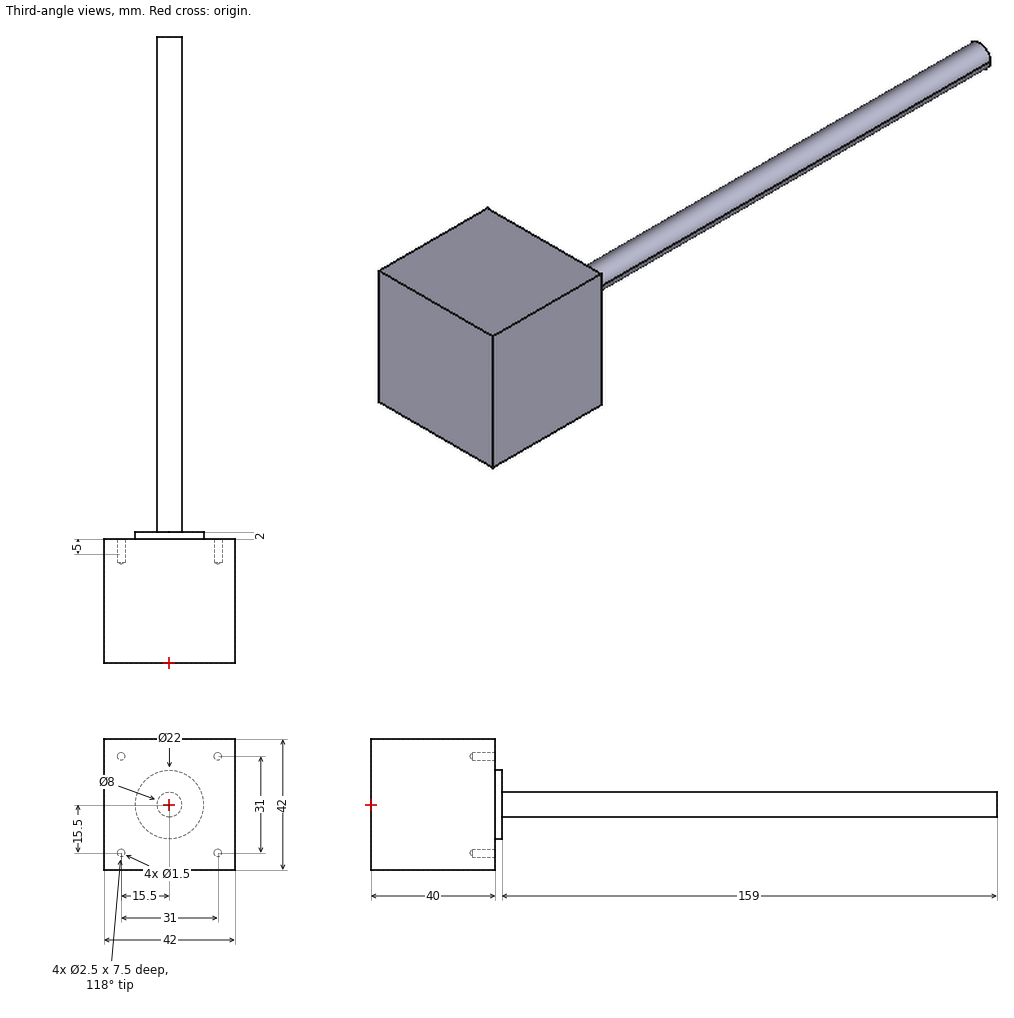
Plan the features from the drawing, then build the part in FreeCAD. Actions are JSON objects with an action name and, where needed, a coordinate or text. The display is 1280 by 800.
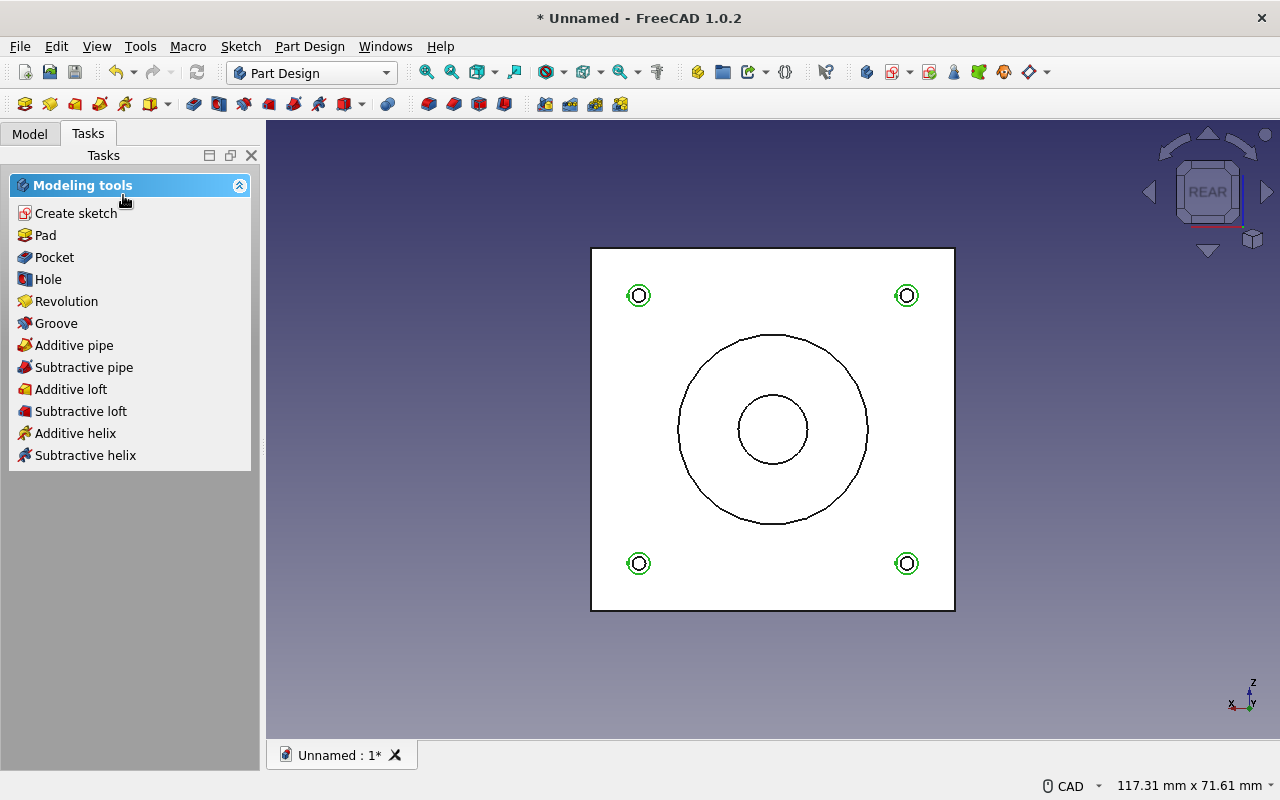
{"action": "left_click", "coordinate": [219, 104]}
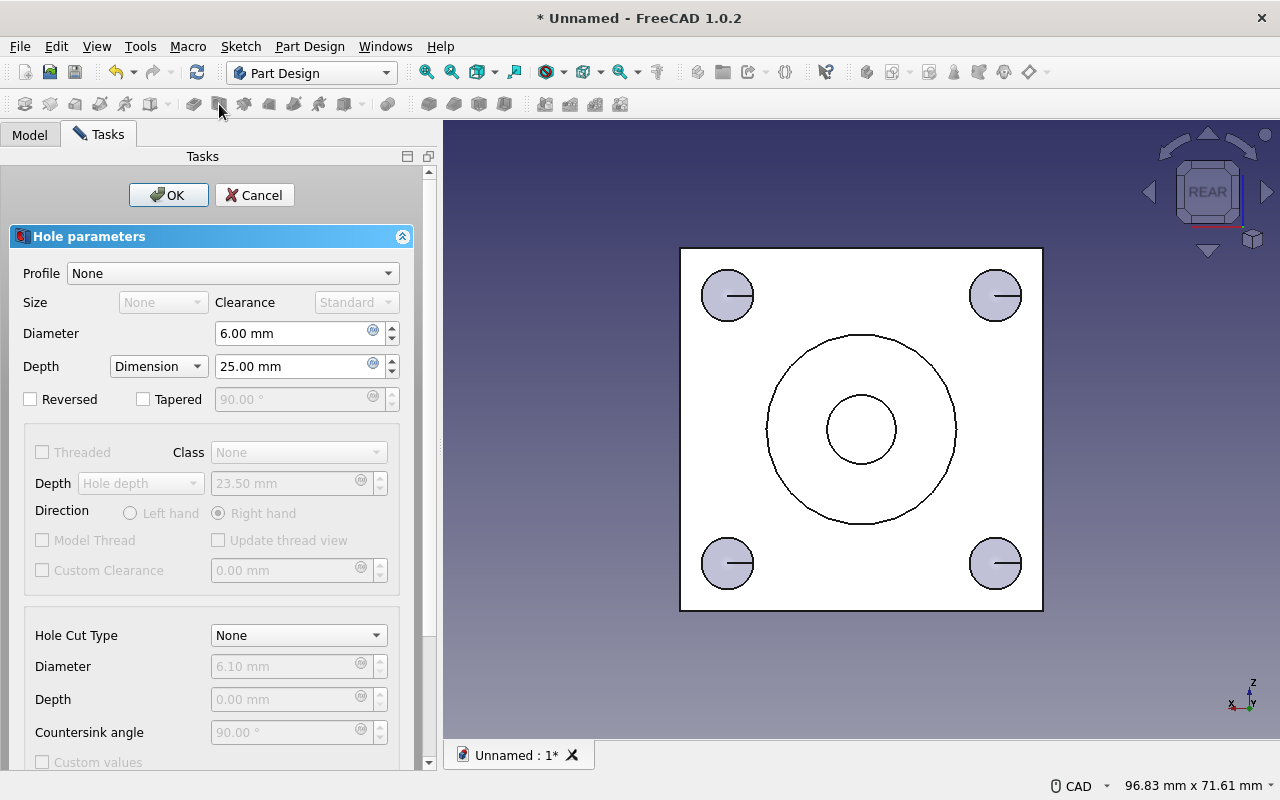
{"action": "triple_click", "coordinate": [300, 334]}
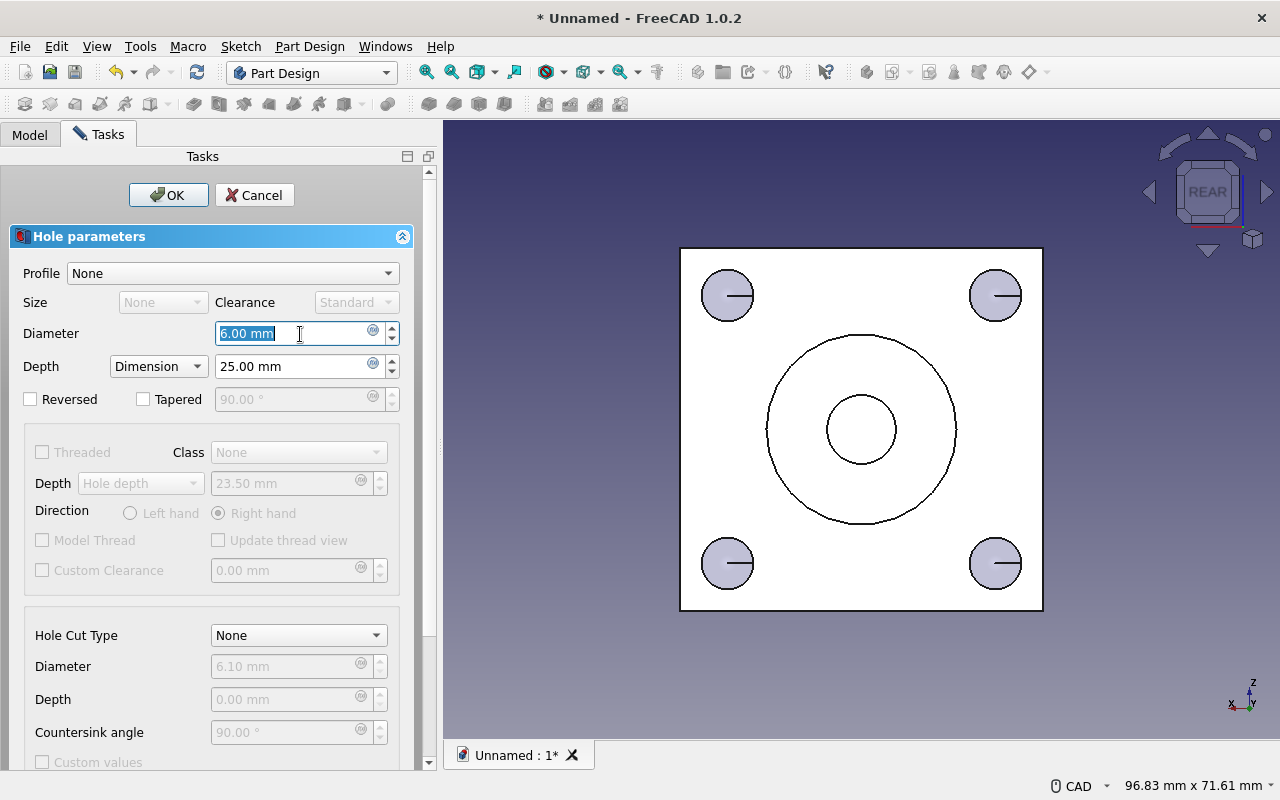
{"action": "type", "text": "2.5"}
{"action": "key", "text": "Tab"}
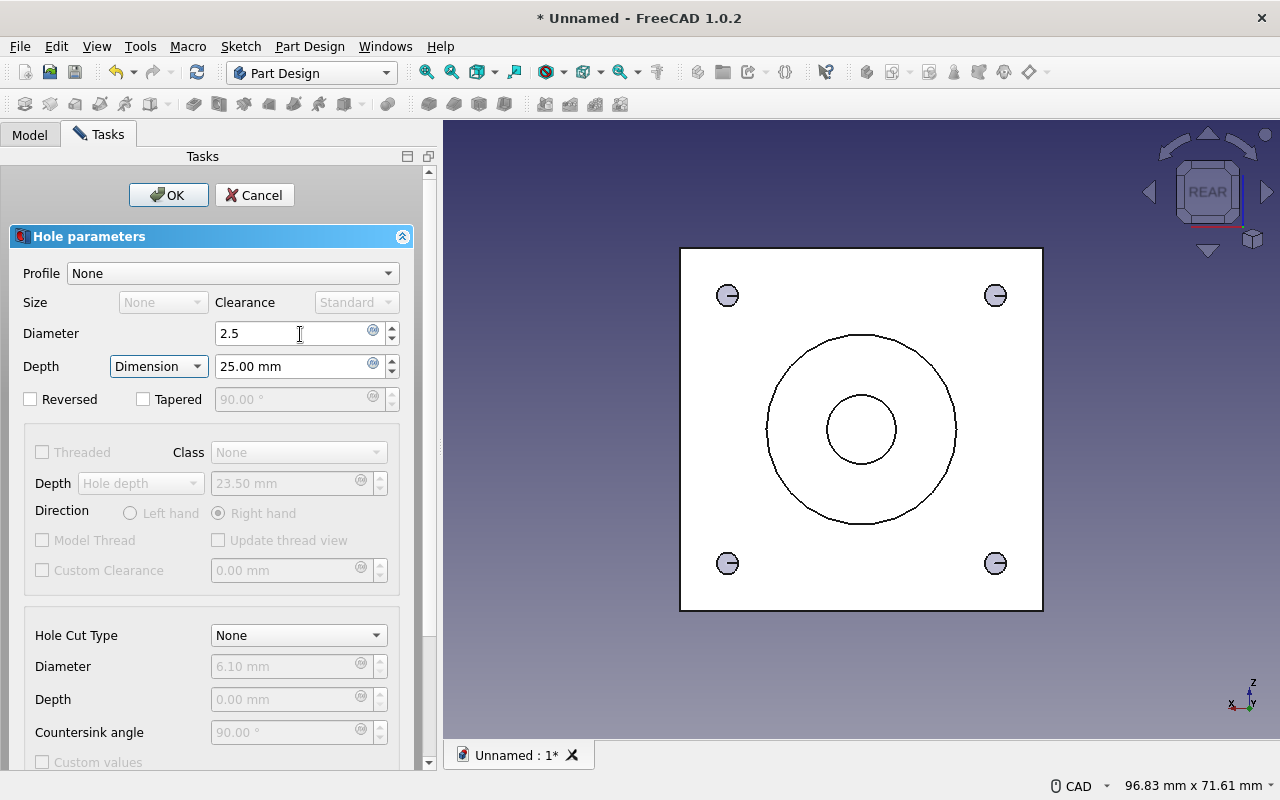
{"action": "triple_click", "coordinate": [300, 366]}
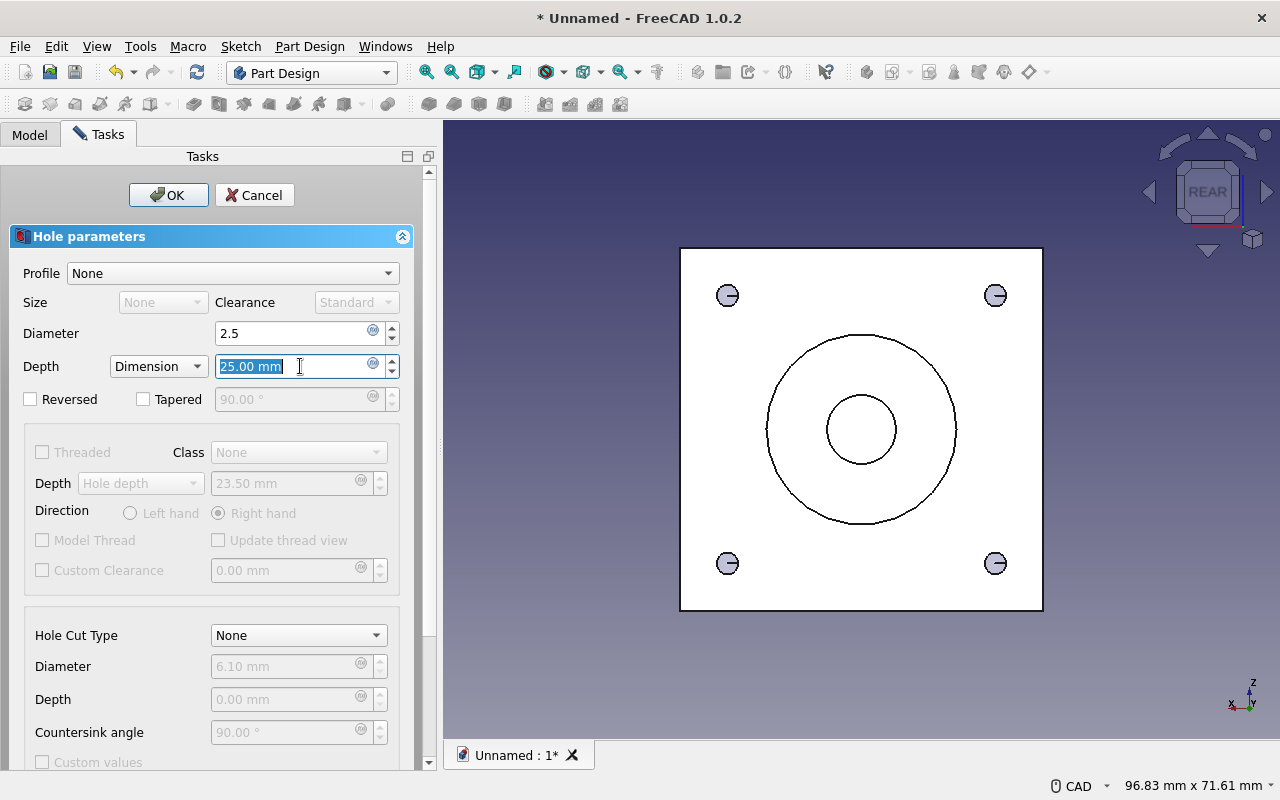
{"action": "type", "text": "7.5"}
{"action": "key", "text": "Tab"}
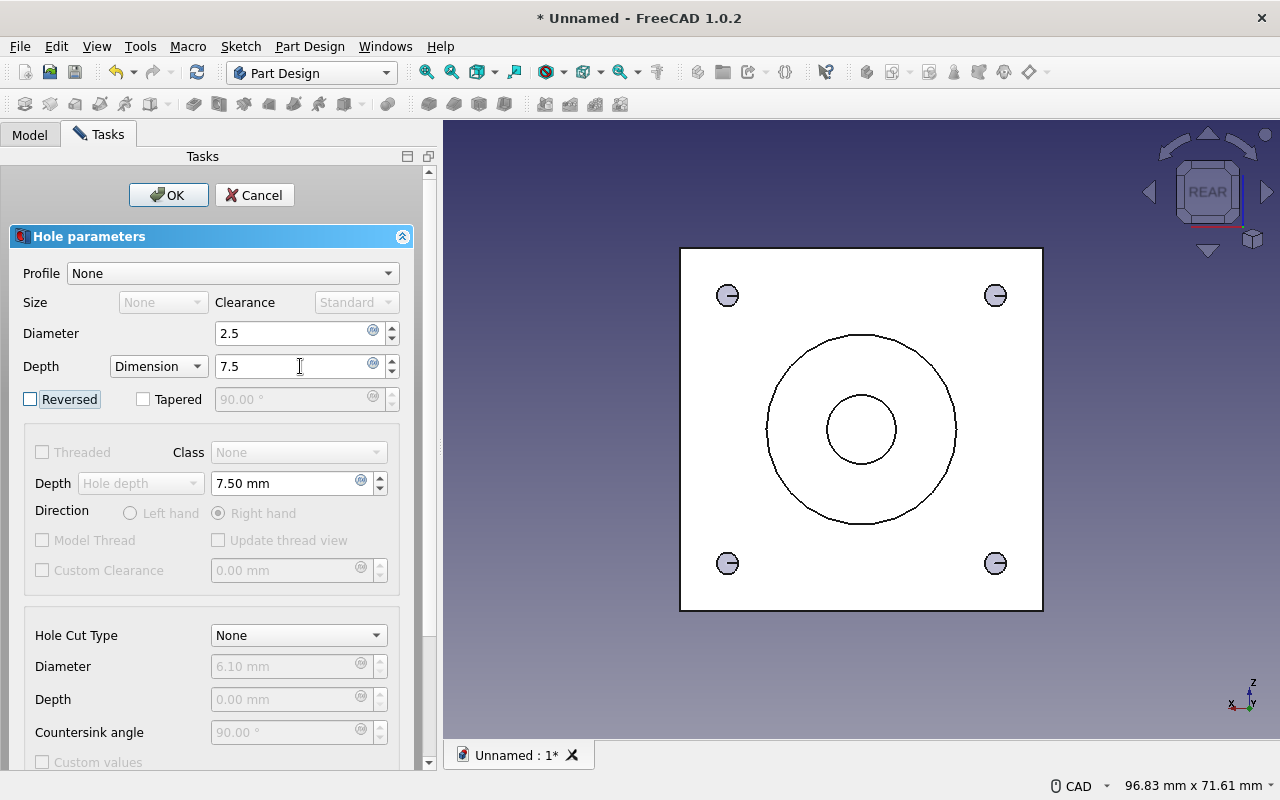
{"action": "left_click", "coordinate": [169, 195]}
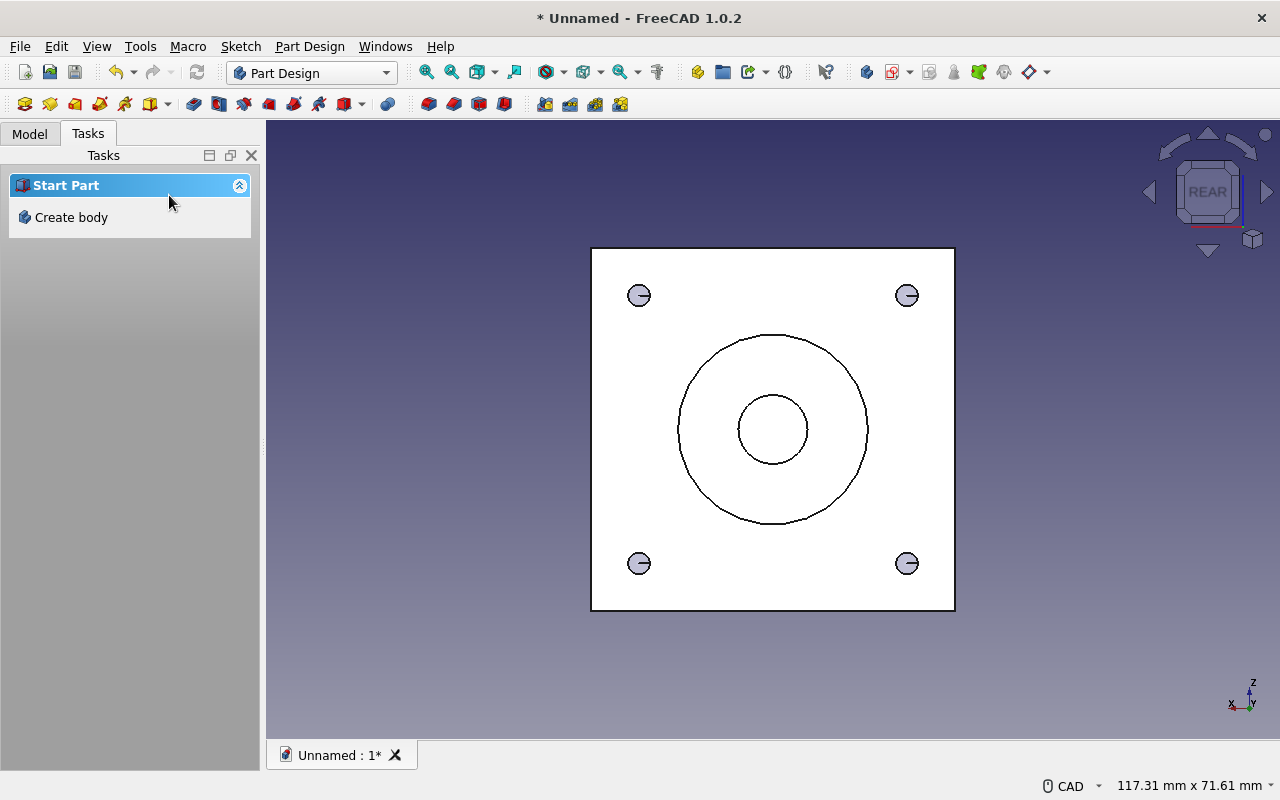
{"action": "key", "text": "0"}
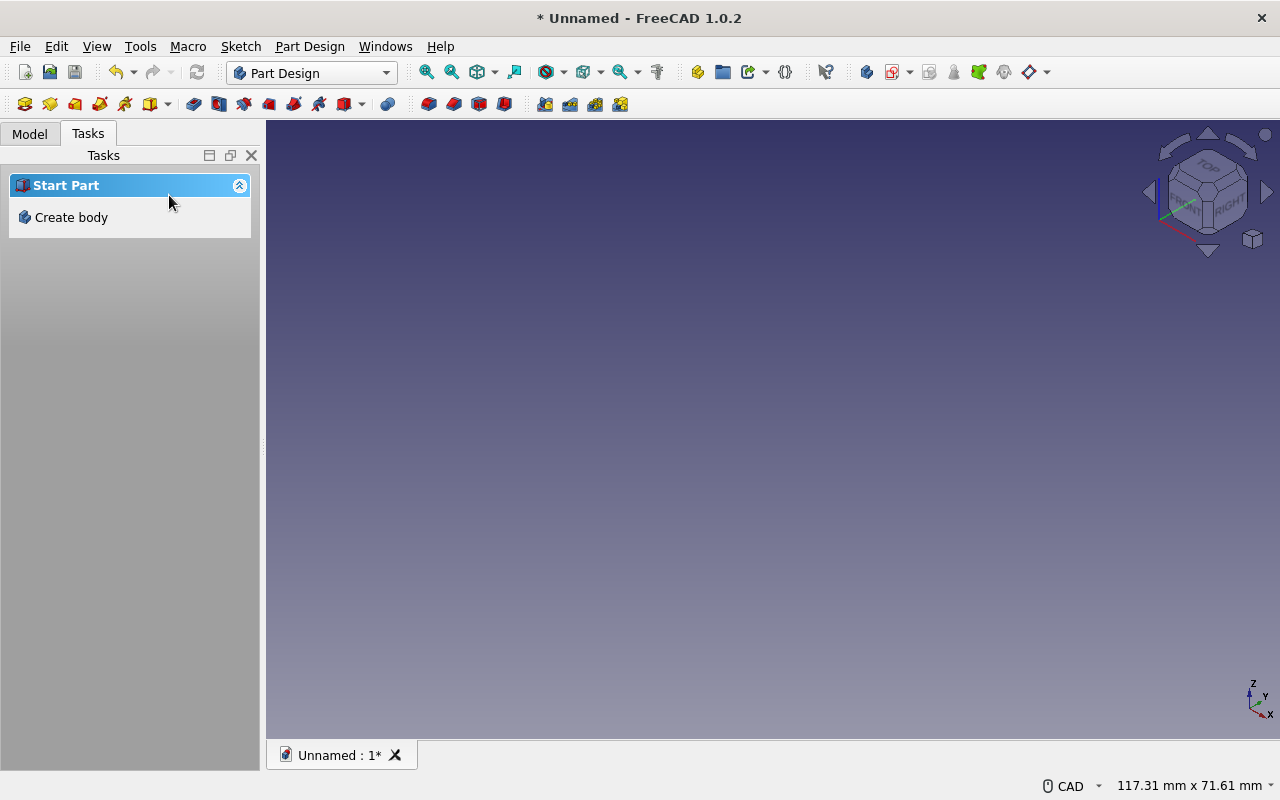
{"action": "left_click", "coordinate": [427, 72]}